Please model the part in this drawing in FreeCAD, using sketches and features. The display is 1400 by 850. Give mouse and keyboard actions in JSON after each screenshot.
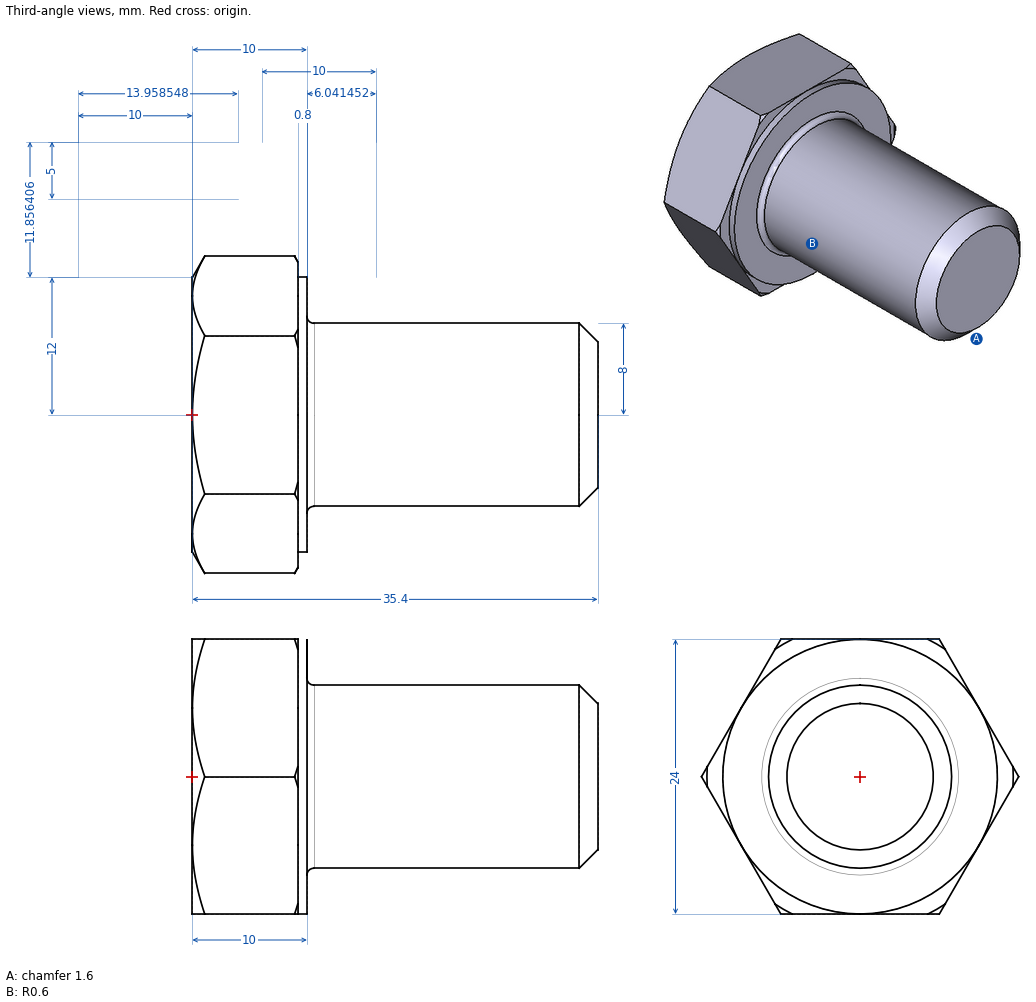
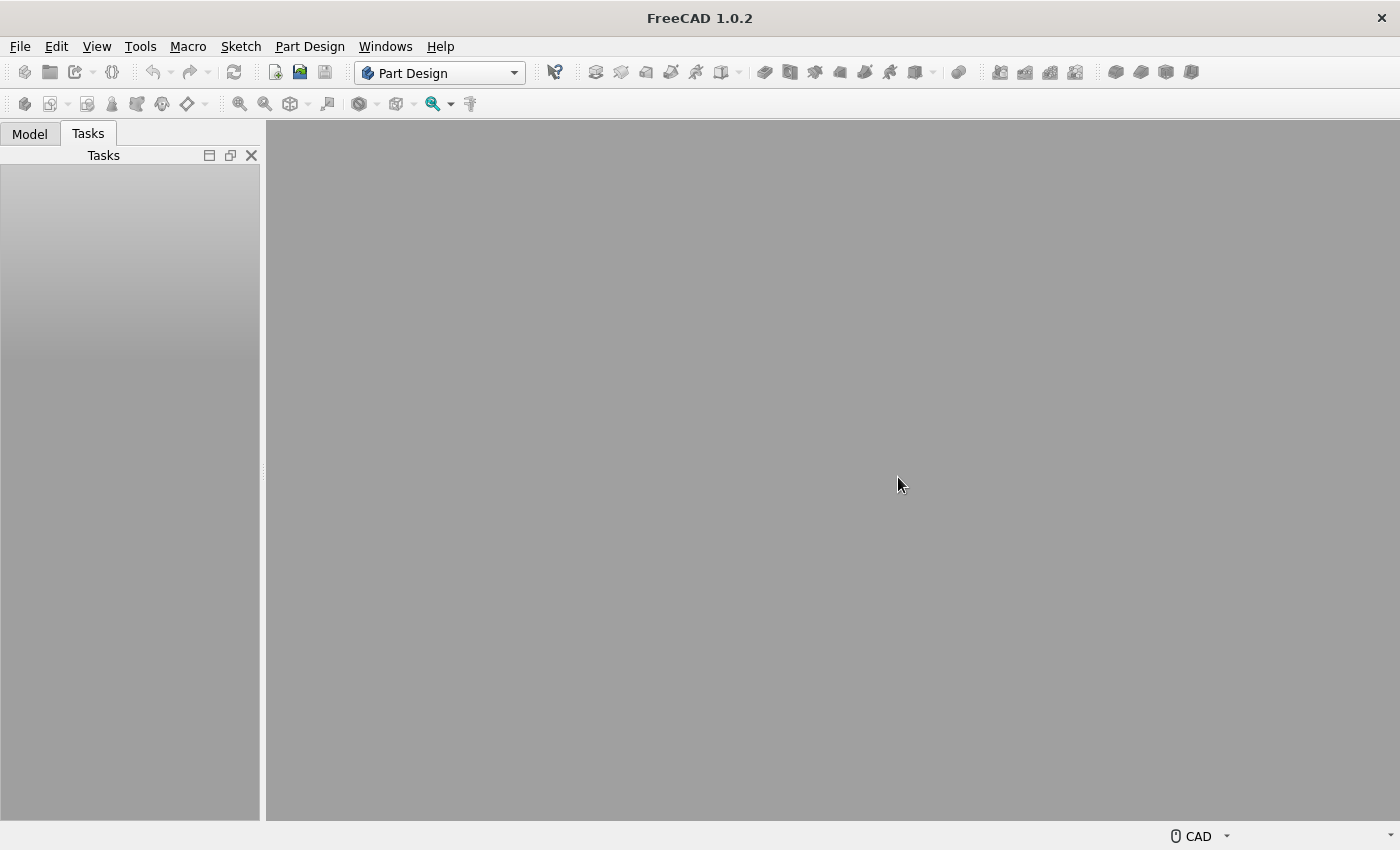
{"action": "key", "text": "ctrl+n"}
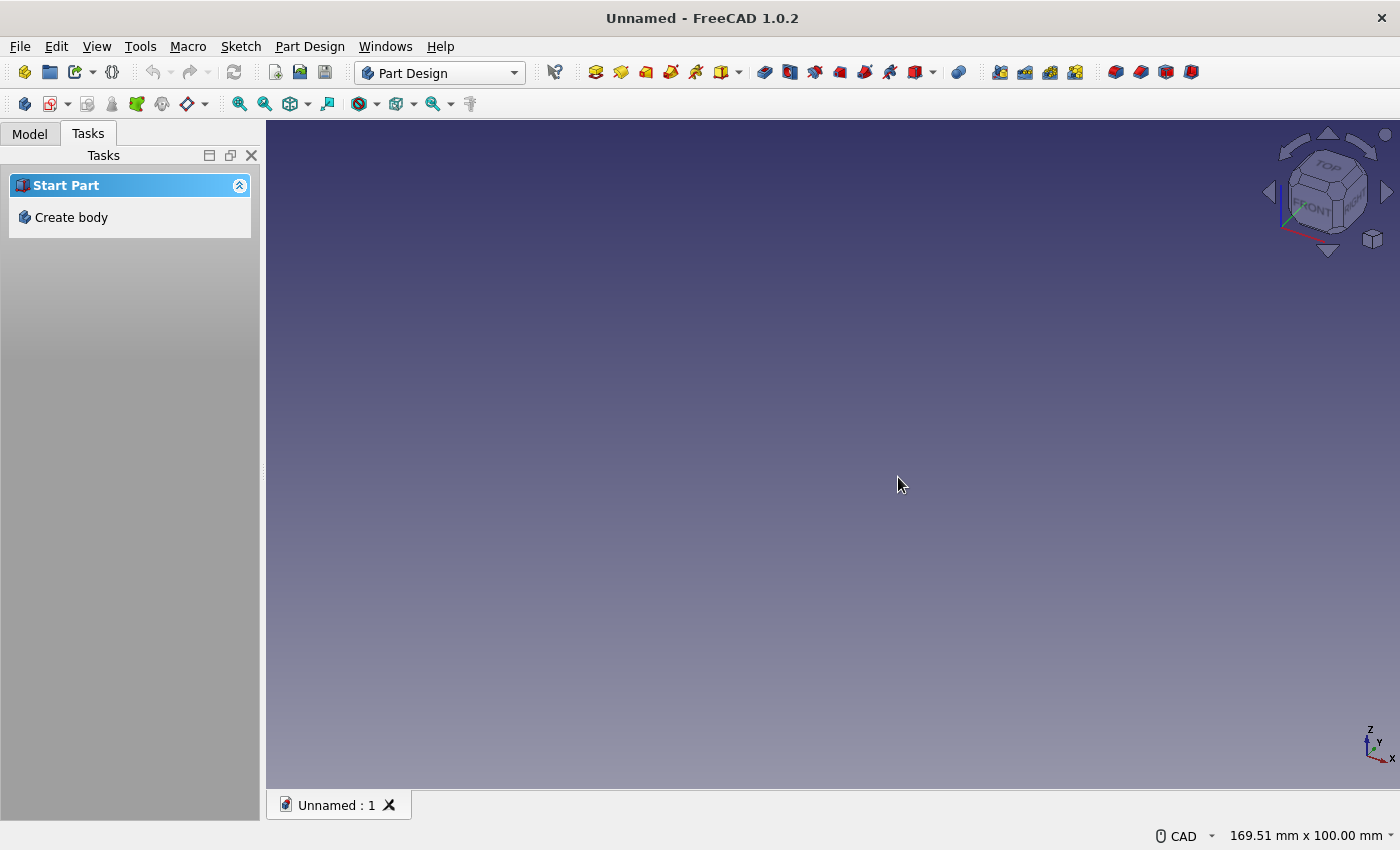
{"action": "left_click", "coordinate": [50, 104]}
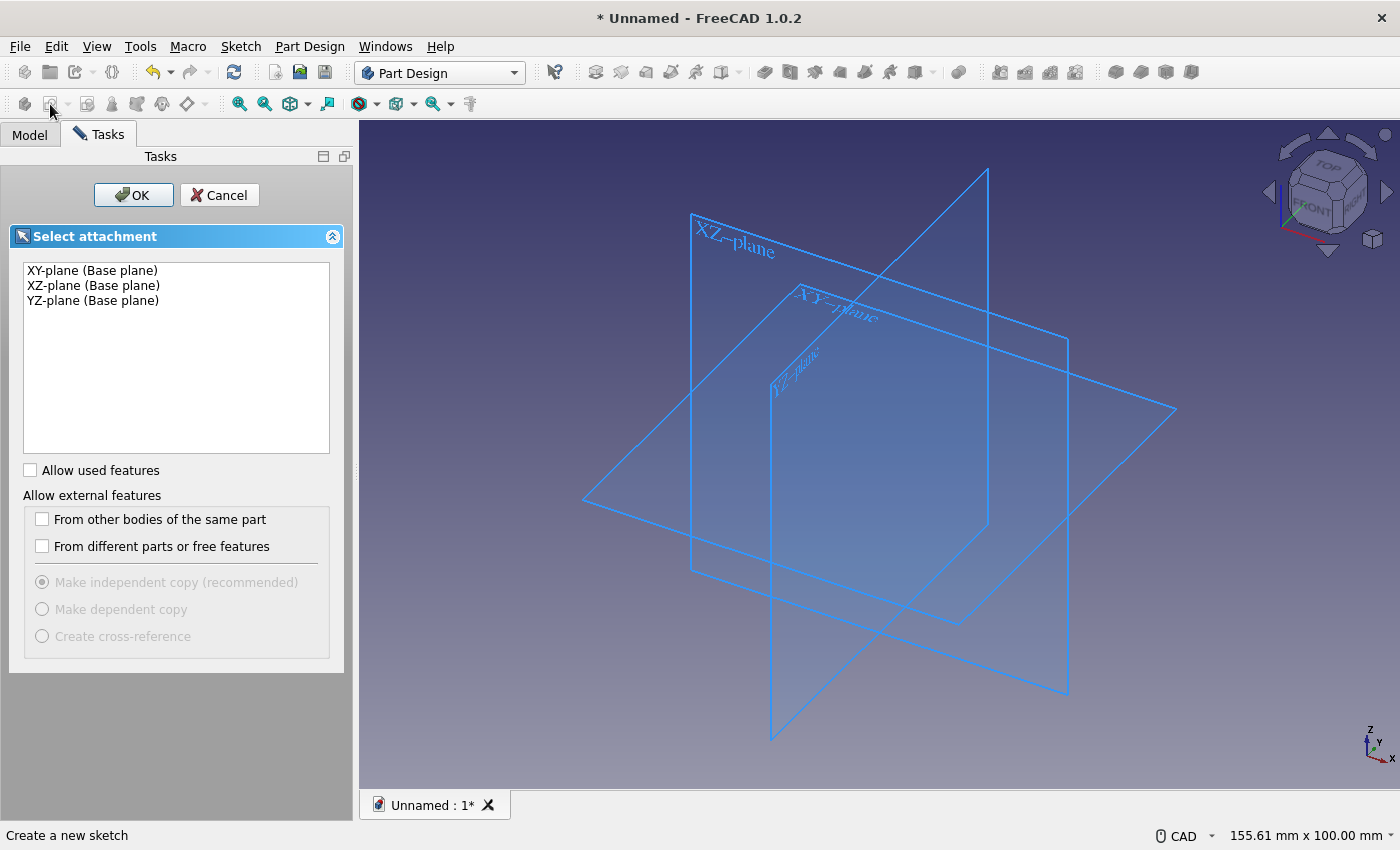
{"action": "left_click", "coordinate": [84, 300]}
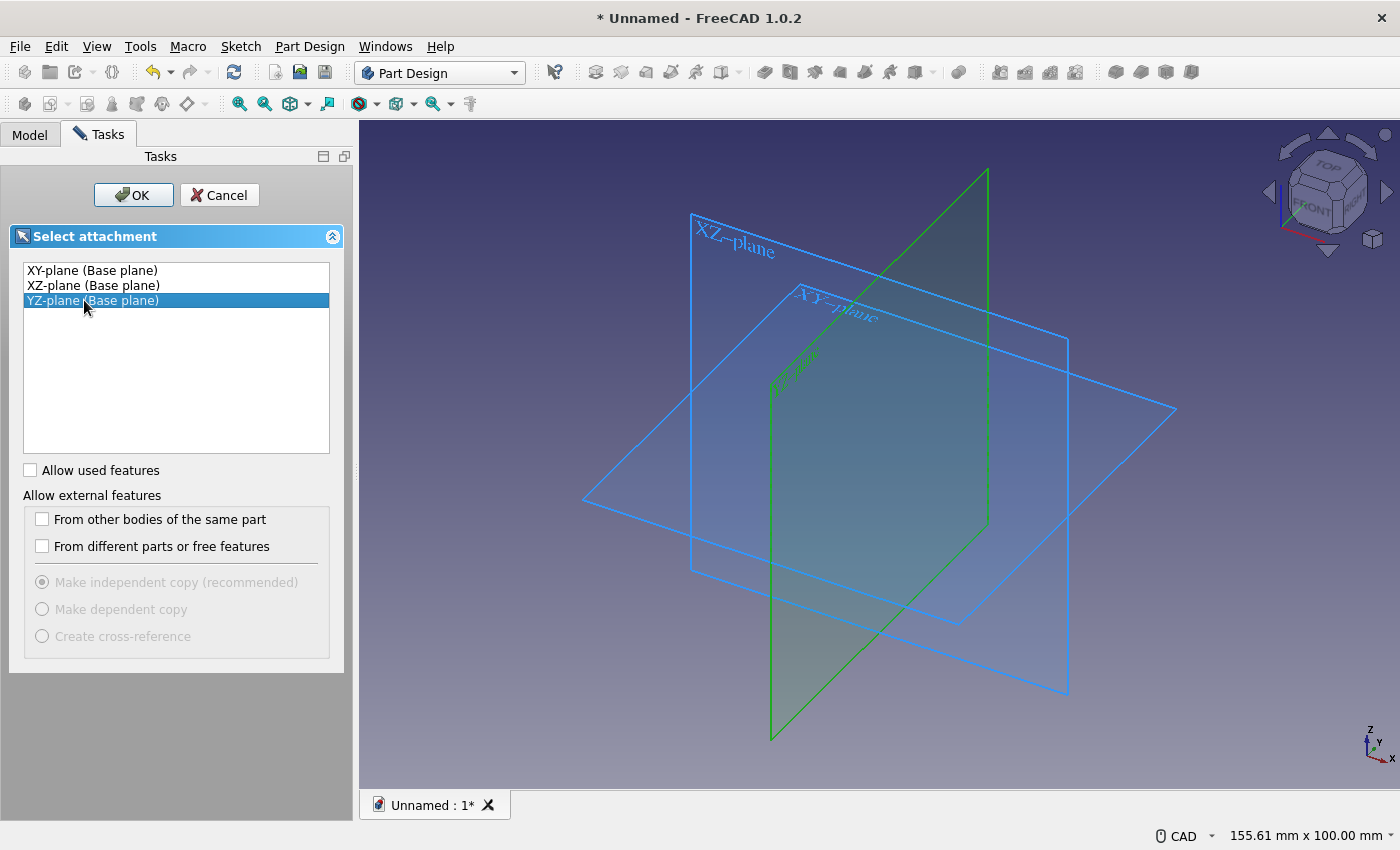
{"action": "left_click", "coordinate": [134, 195]}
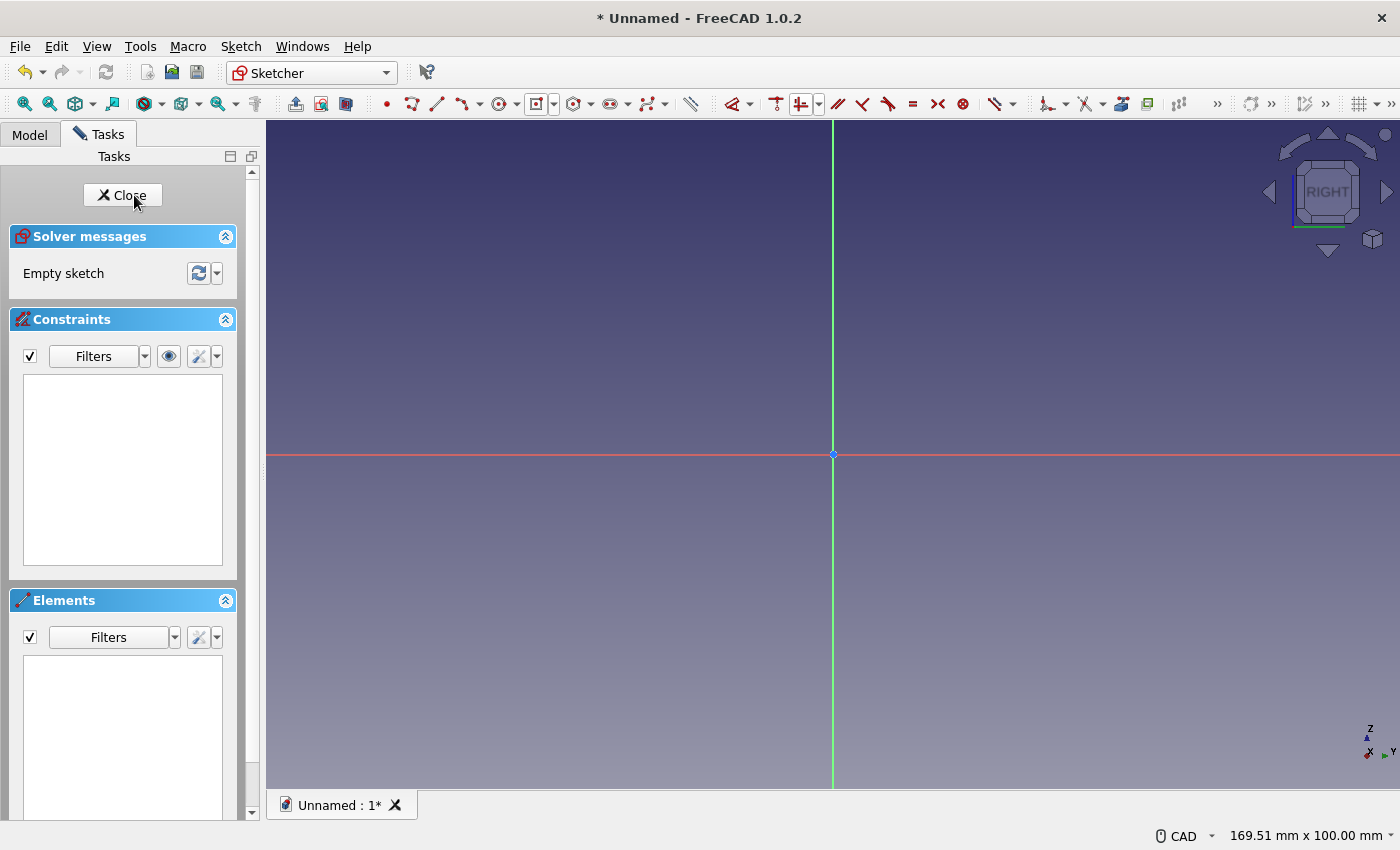
{"action": "scroll", "coordinate": [873, 454], "scroll_direction": "up", "scroll_amount": 5}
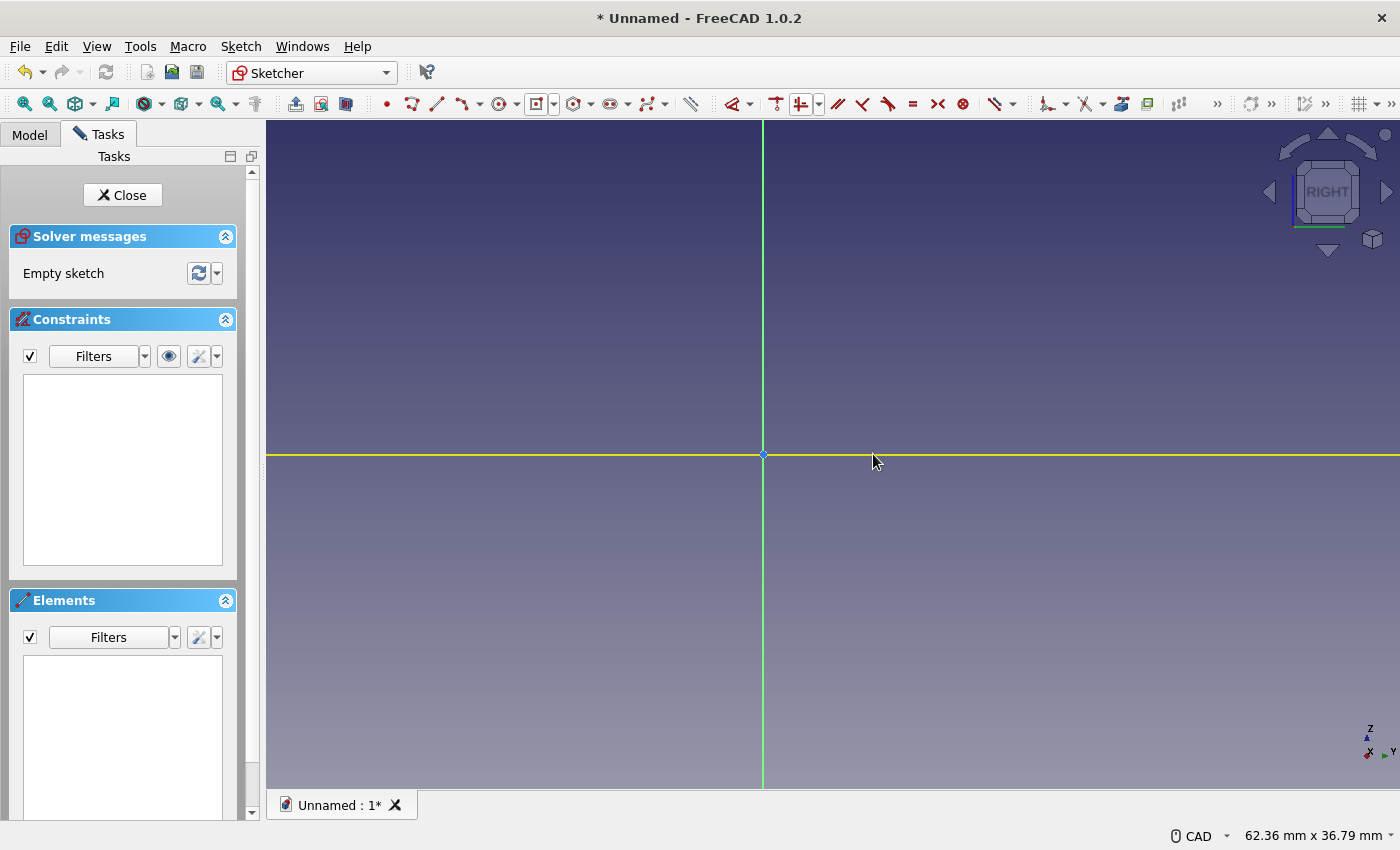
{"action": "key", "text": "g p 6"}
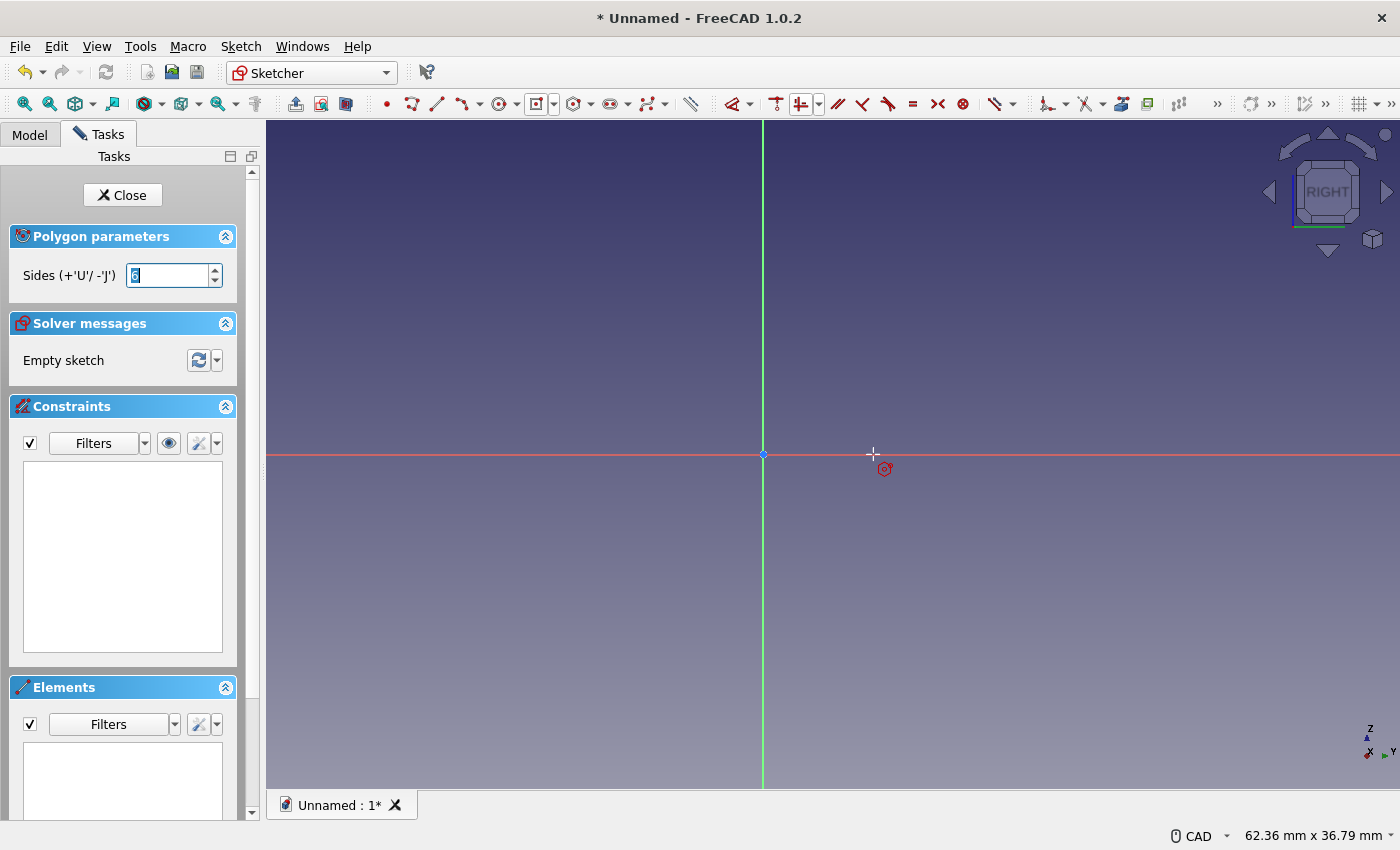
{"action": "left_click", "coordinate": [763, 454]}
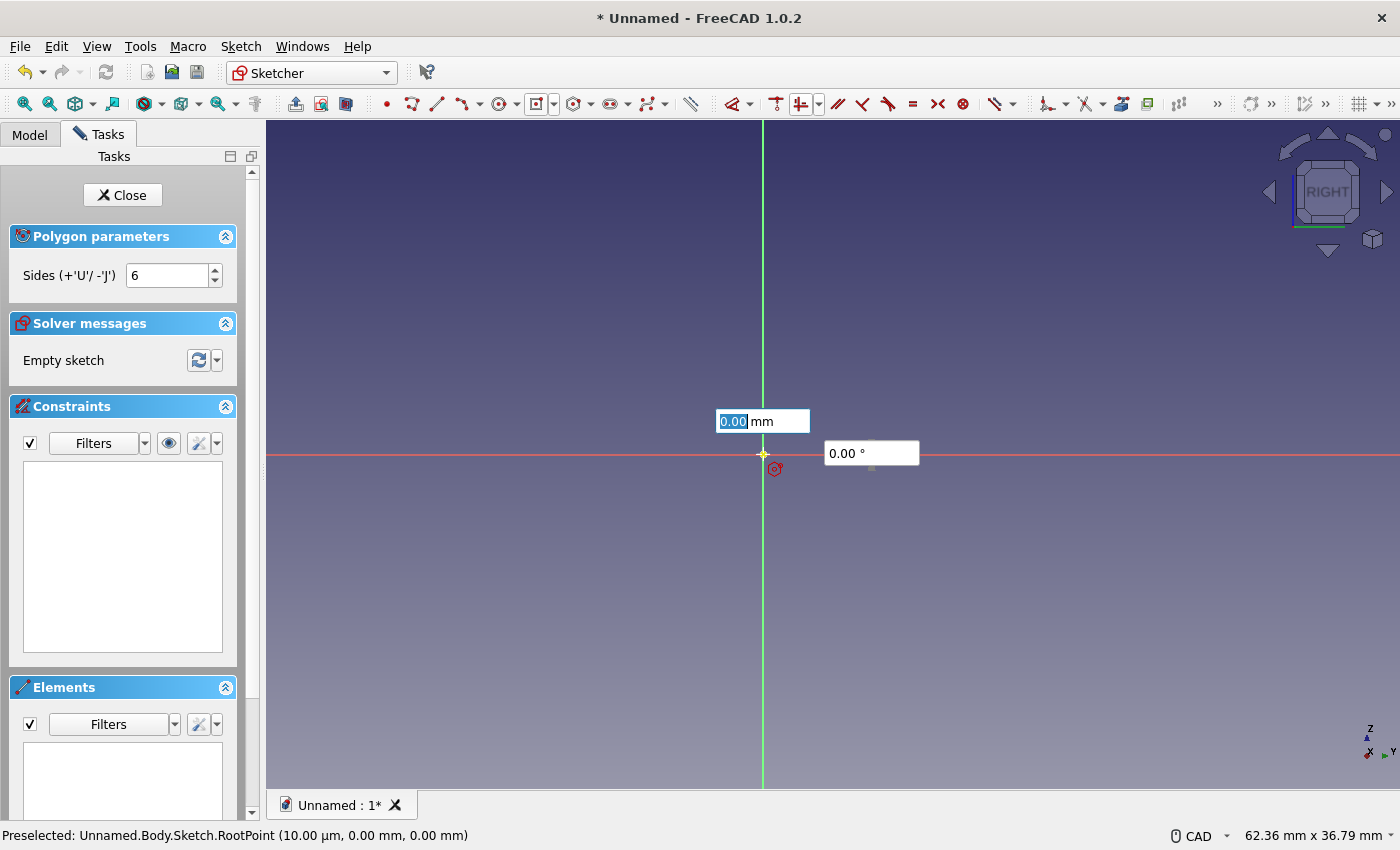
{"action": "left_click", "coordinate": [1015, 454]}
{"action": "right_click", "coordinate": [1015, 454]}